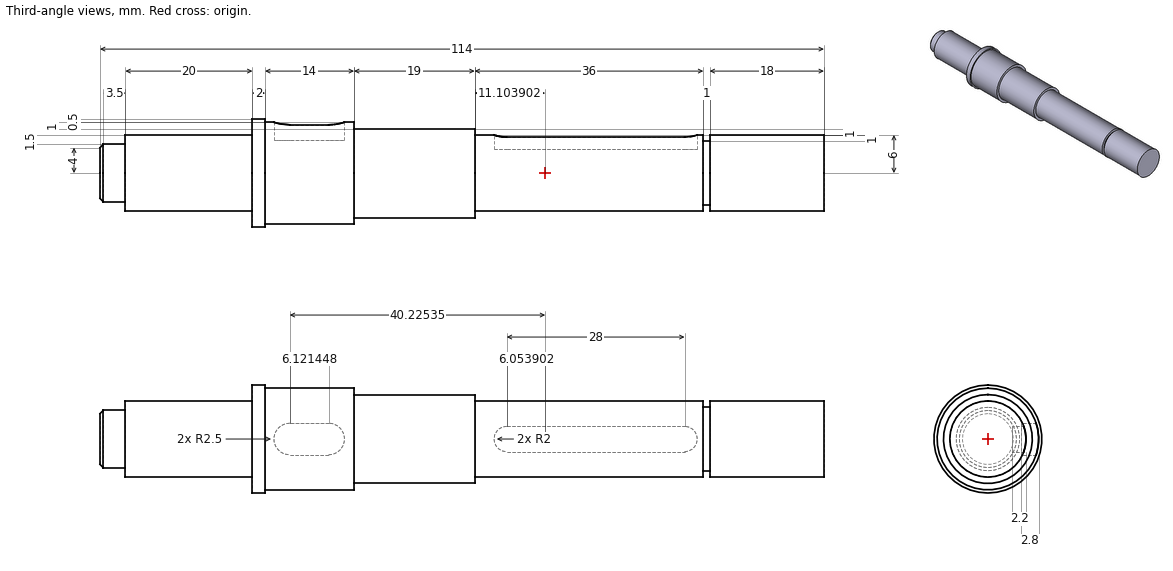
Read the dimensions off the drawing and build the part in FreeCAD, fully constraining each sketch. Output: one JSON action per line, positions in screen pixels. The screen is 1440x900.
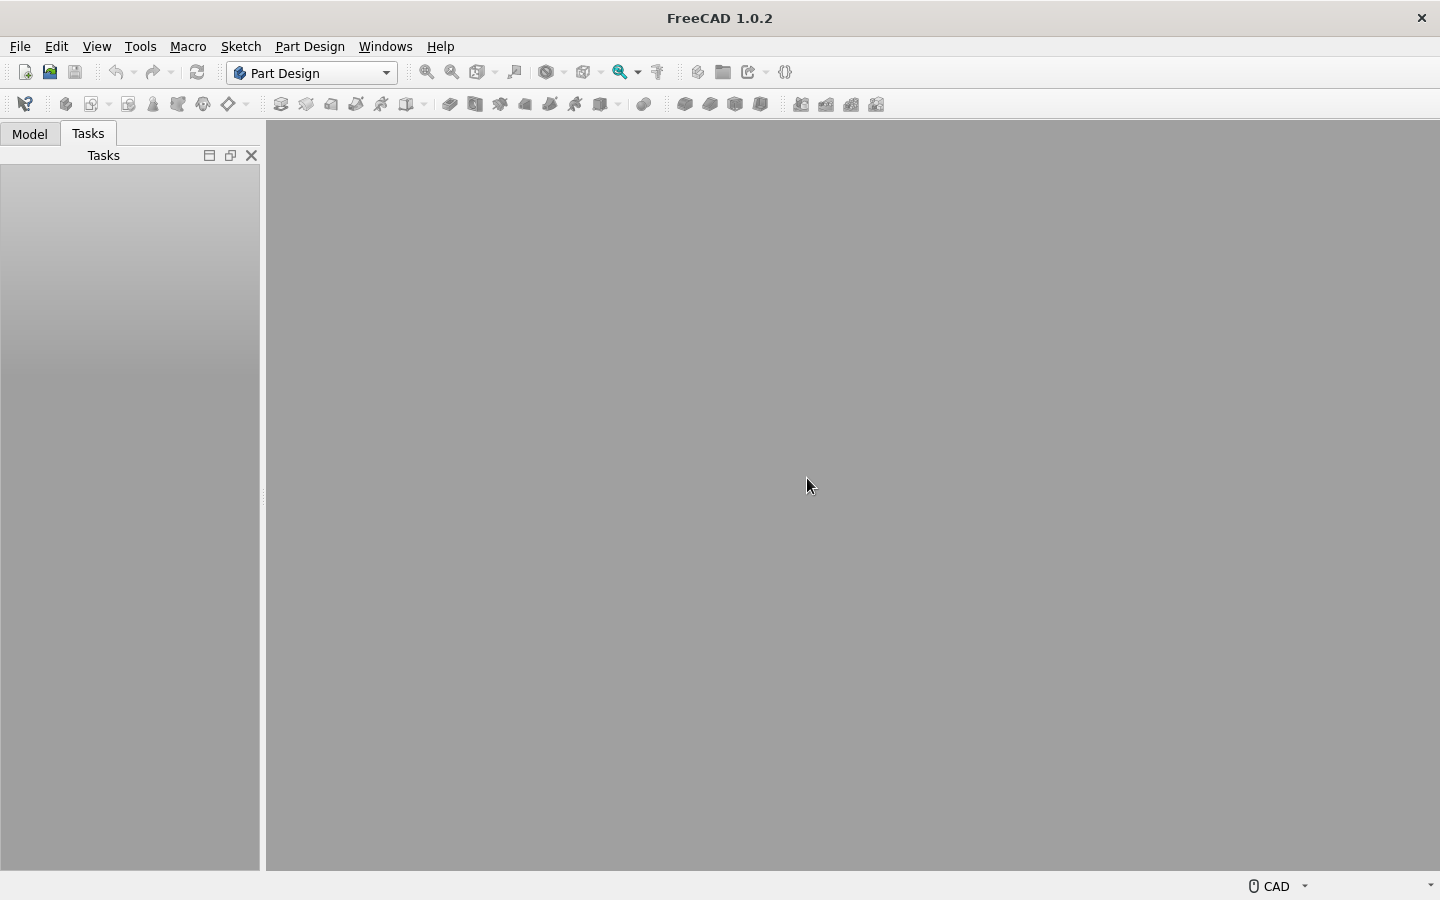
{"action": "left_click", "coordinate": [25, 72]}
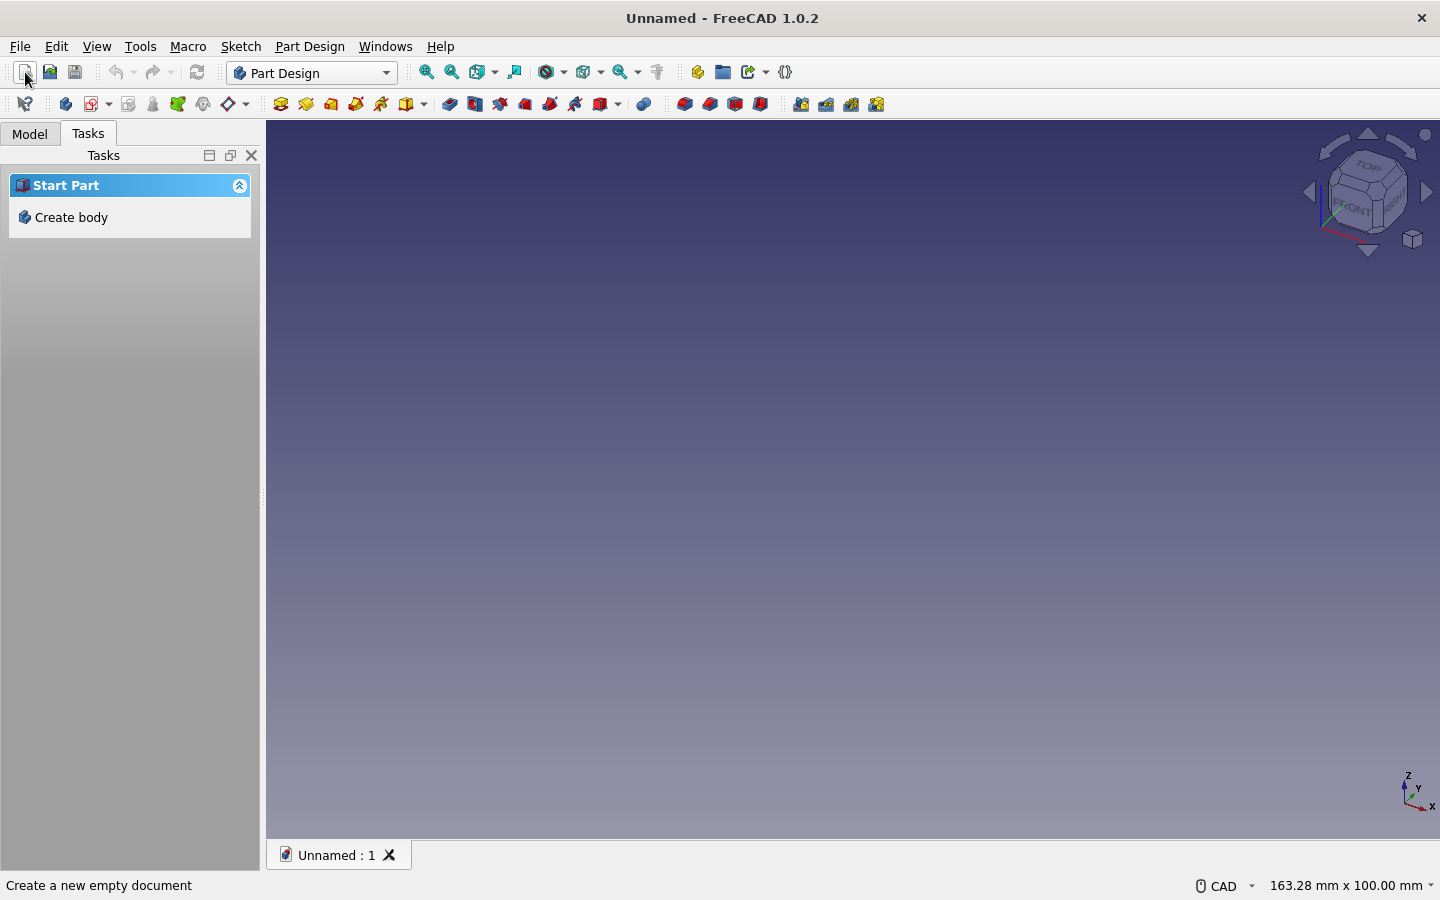
{"action": "left_click", "coordinate": [90, 104]}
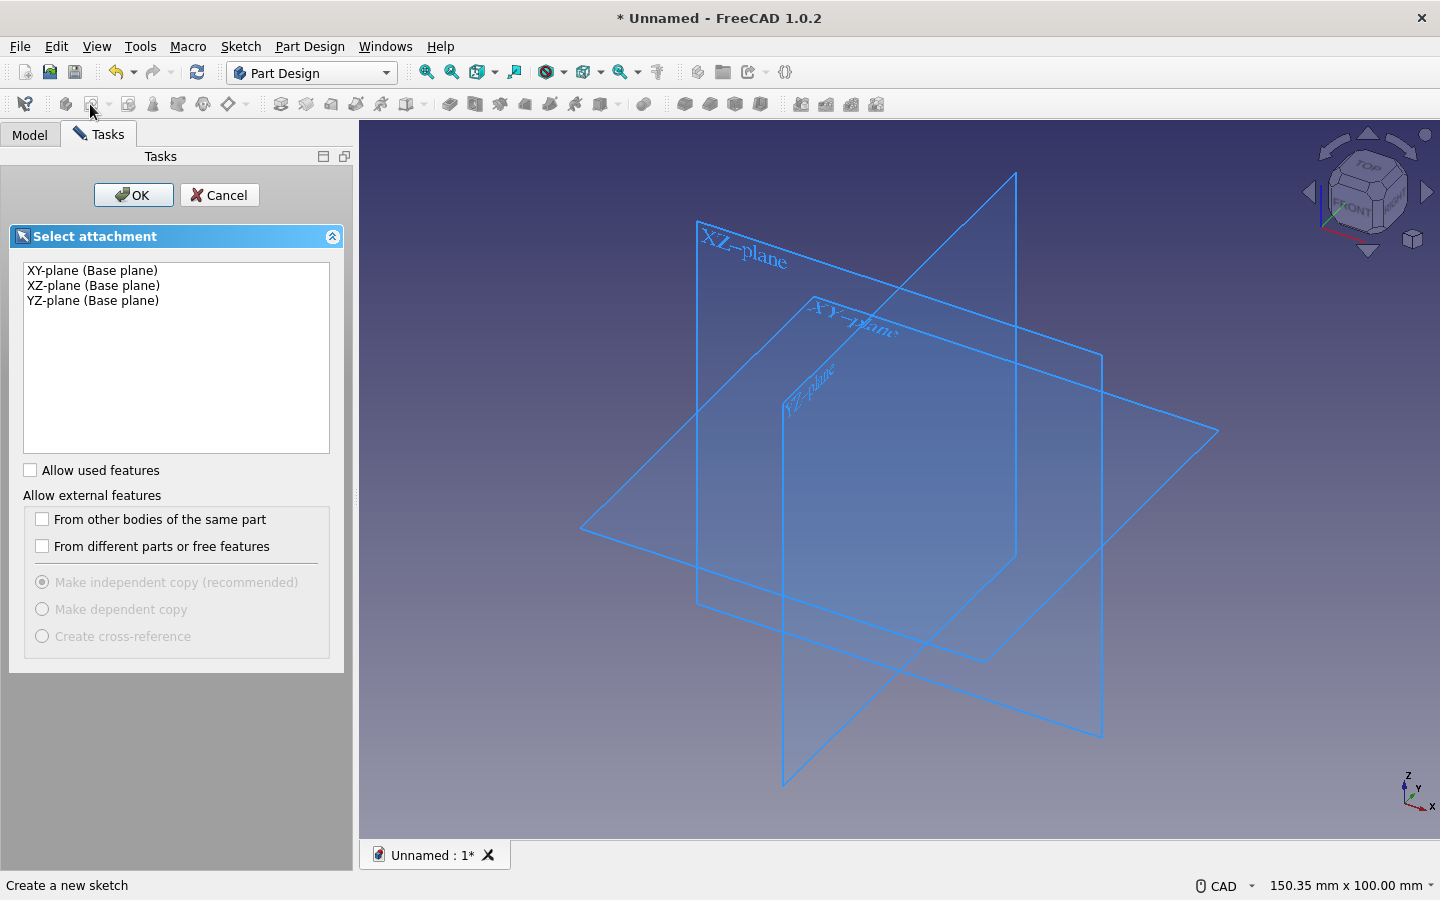
{"action": "left_click", "coordinate": [84, 270]}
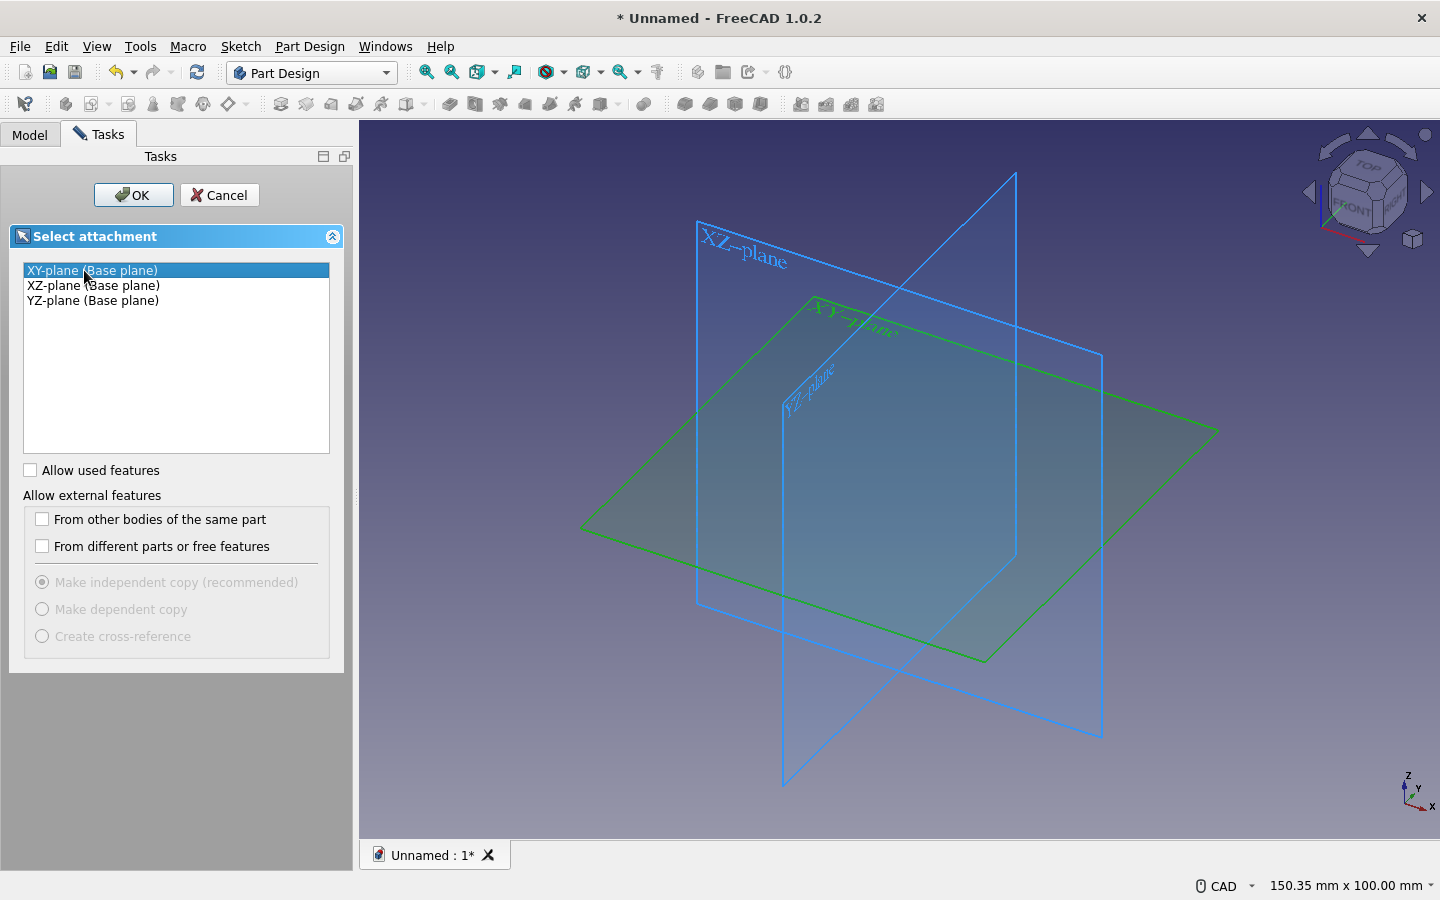
{"action": "left_click", "coordinate": [134, 195]}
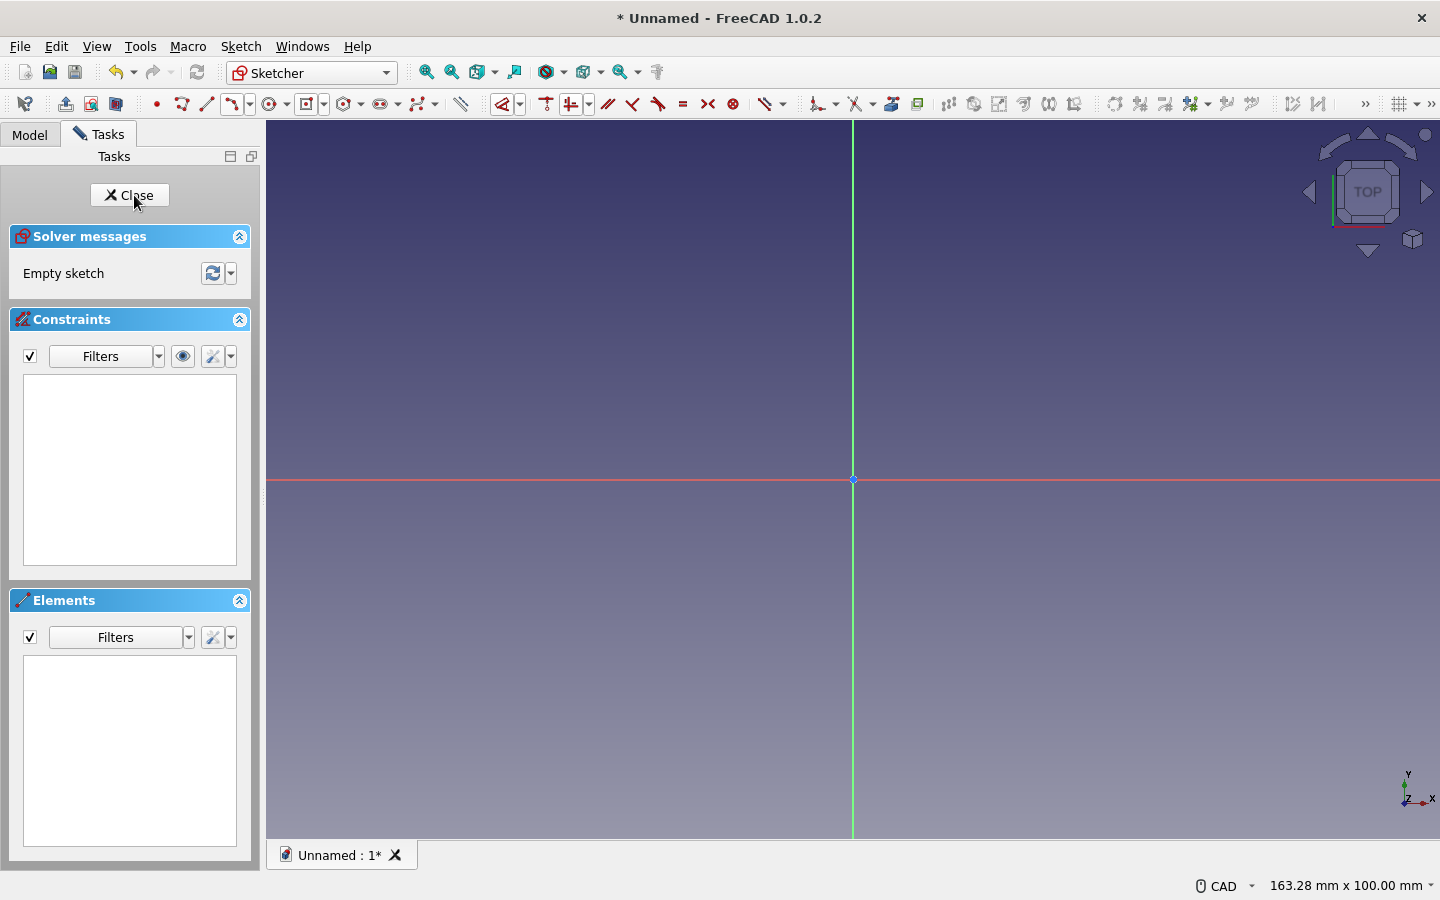
{"action": "key", "text": "g m"}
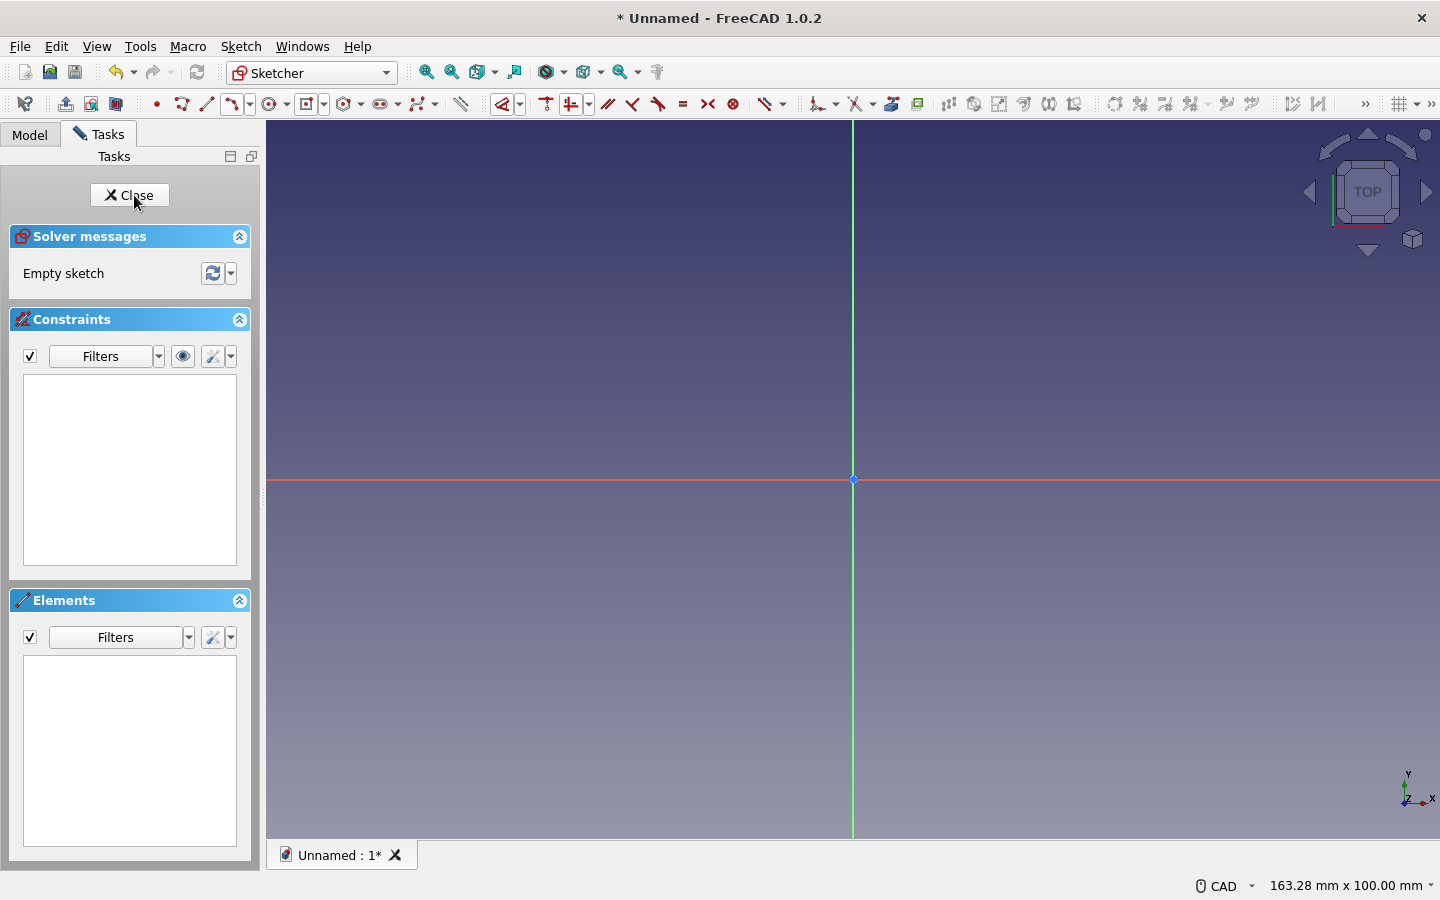
{"action": "left_click", "coordinate": [773, 436]}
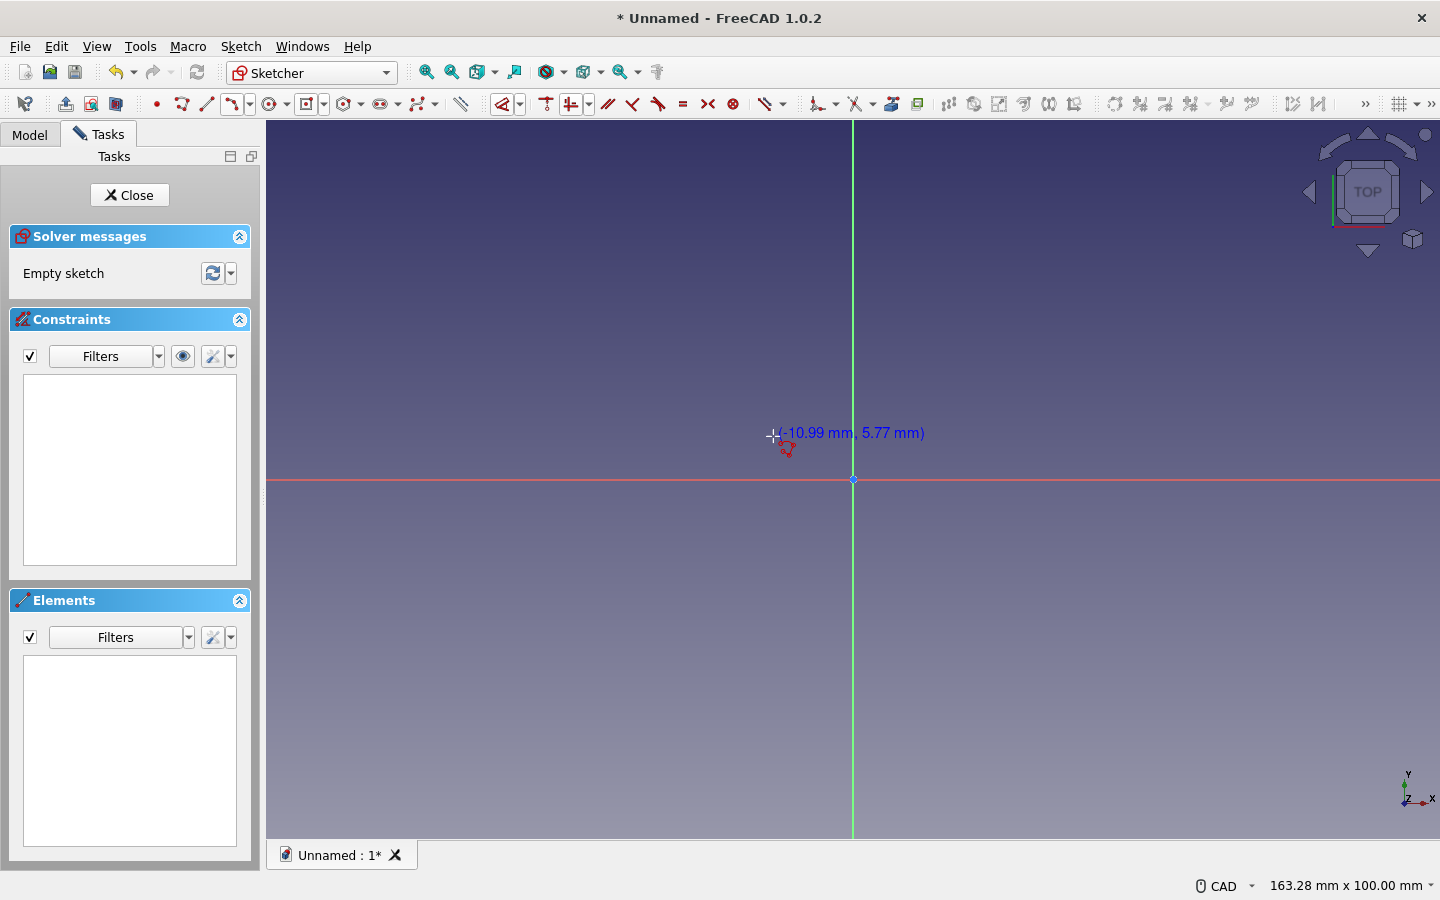
{"action": "scroll", "coordinate": [773, 429], "scroll_direction": "up", "scroll_amount": 4}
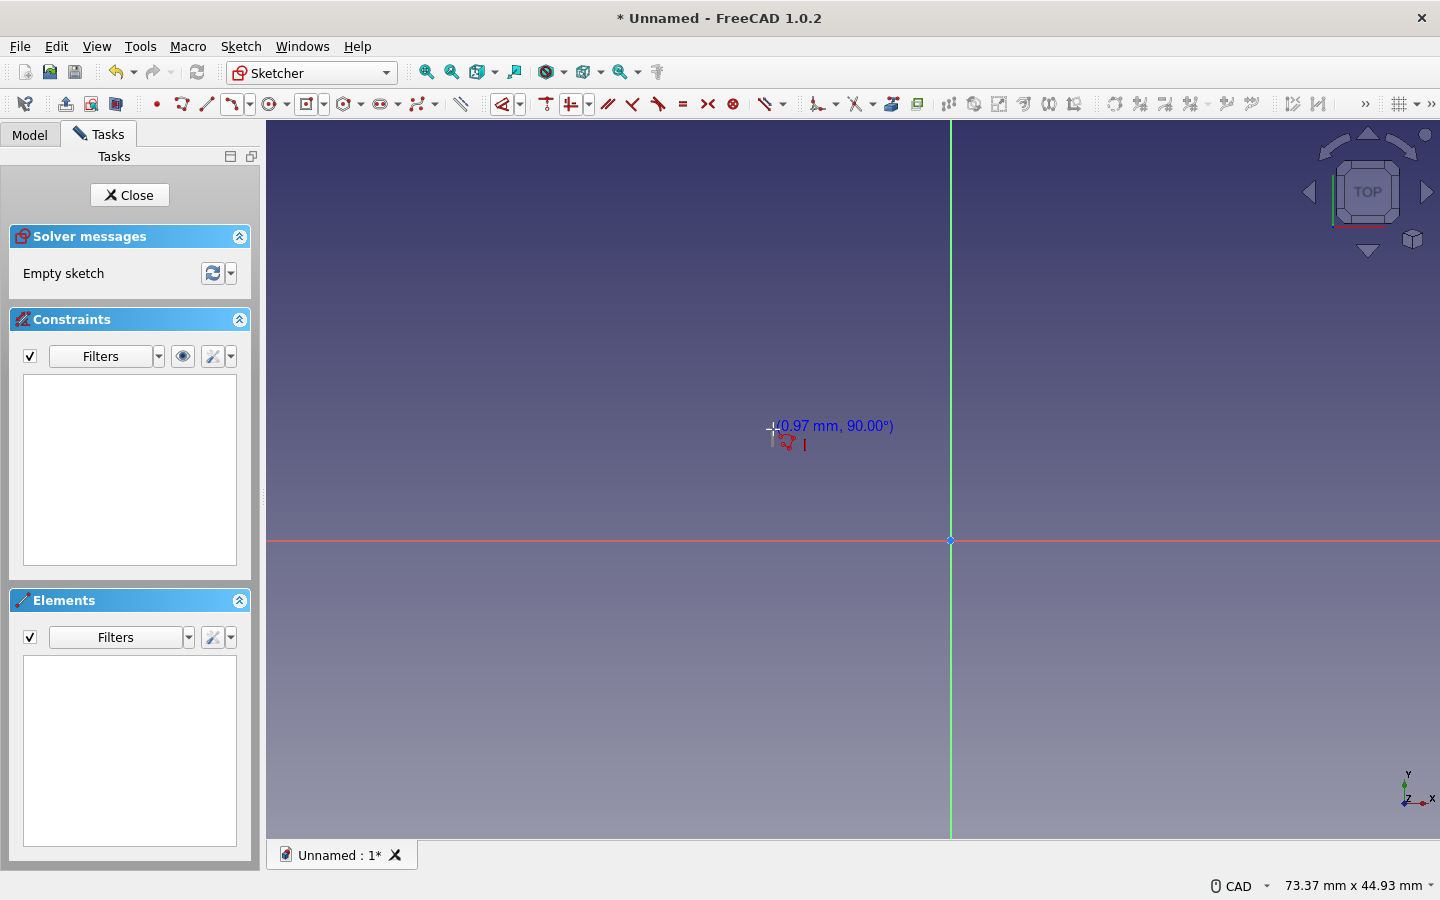
{"action": "left_click", "coordinate": [772, 429]}
{"action": "left_click", "coordinate": [469, 429]}
{"action": "left_click", "coordinate": [469, 413]}